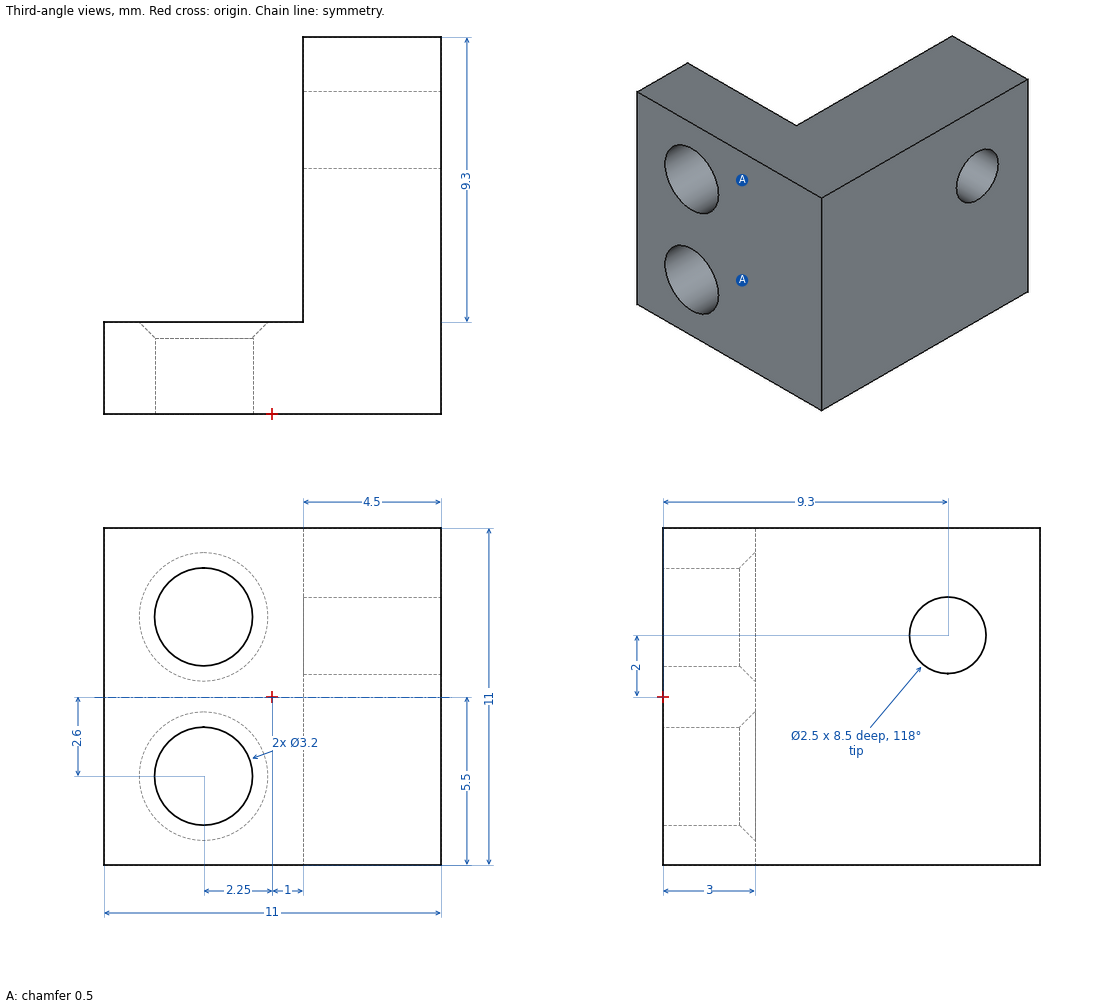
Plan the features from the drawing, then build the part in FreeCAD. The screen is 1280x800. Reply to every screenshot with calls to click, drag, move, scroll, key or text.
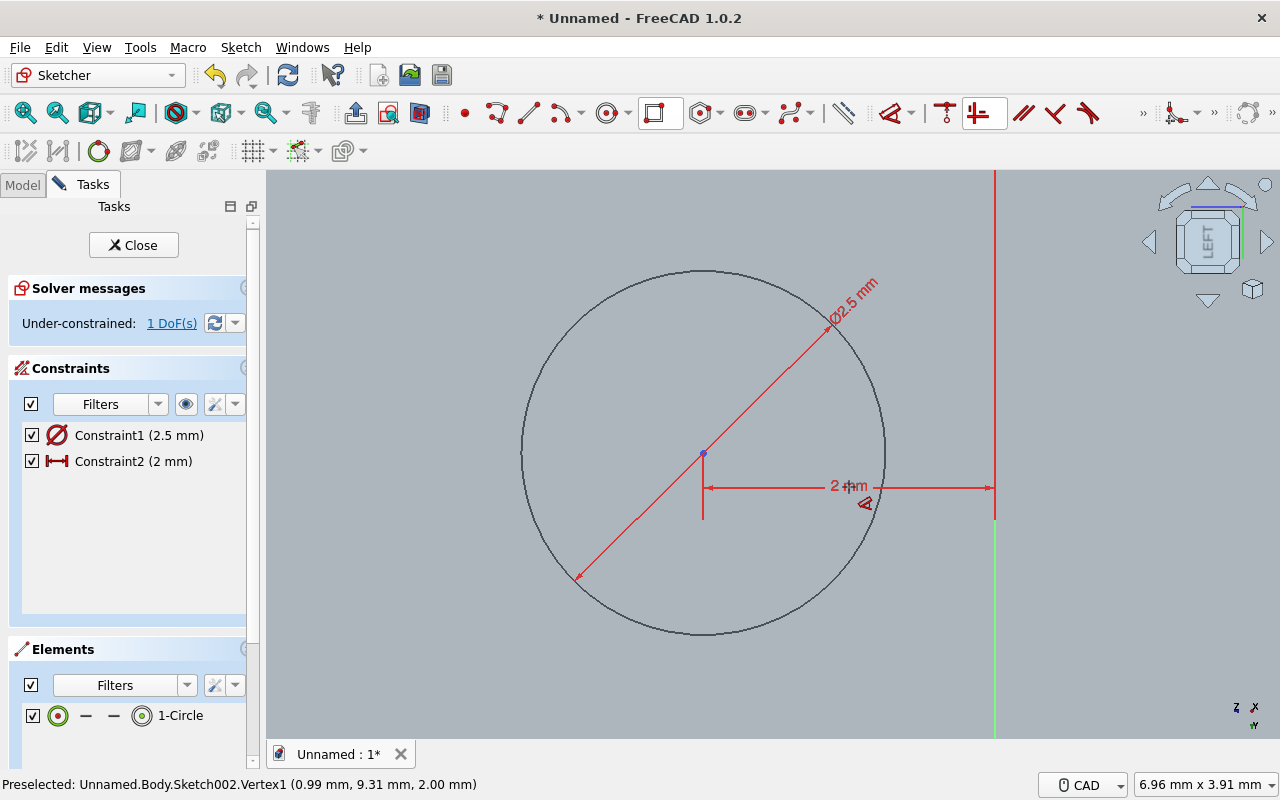
click(703, 453)
click(1029, 326)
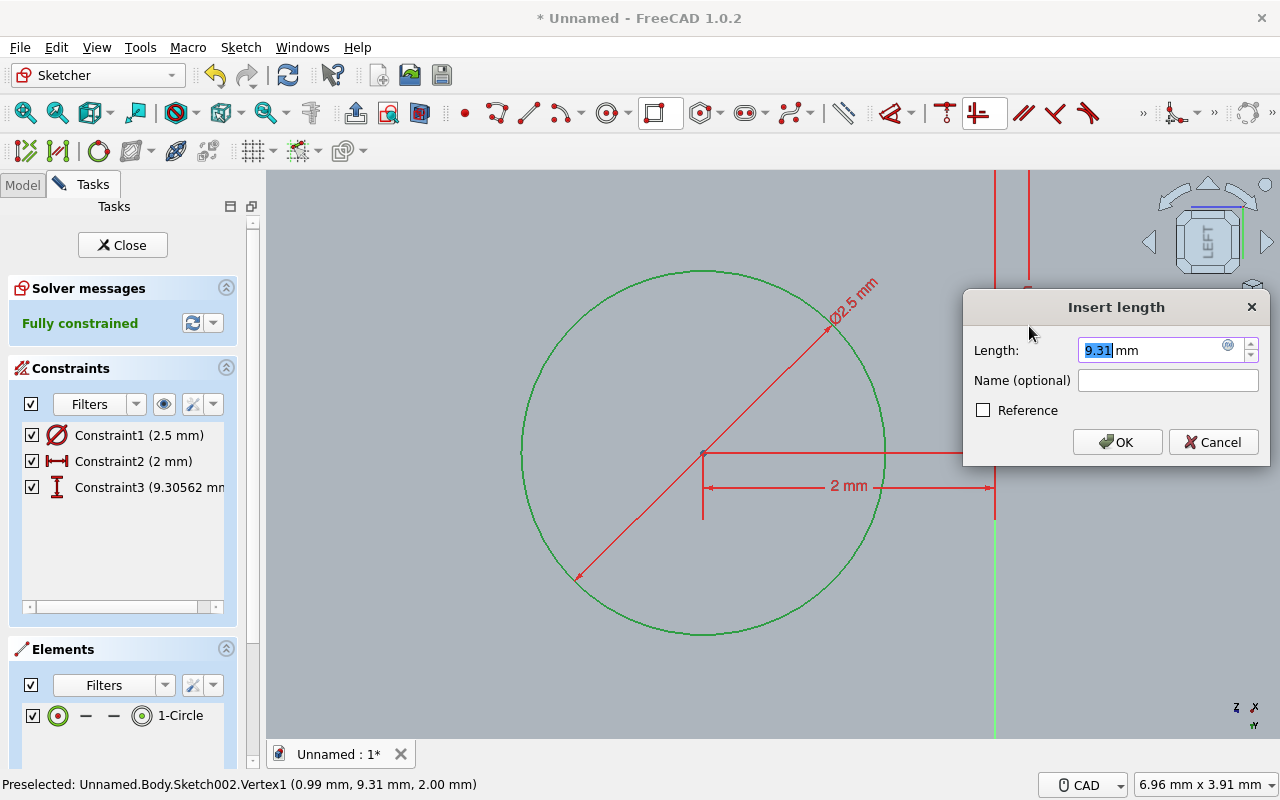
text(9.3)
key(Return)
key(Escape)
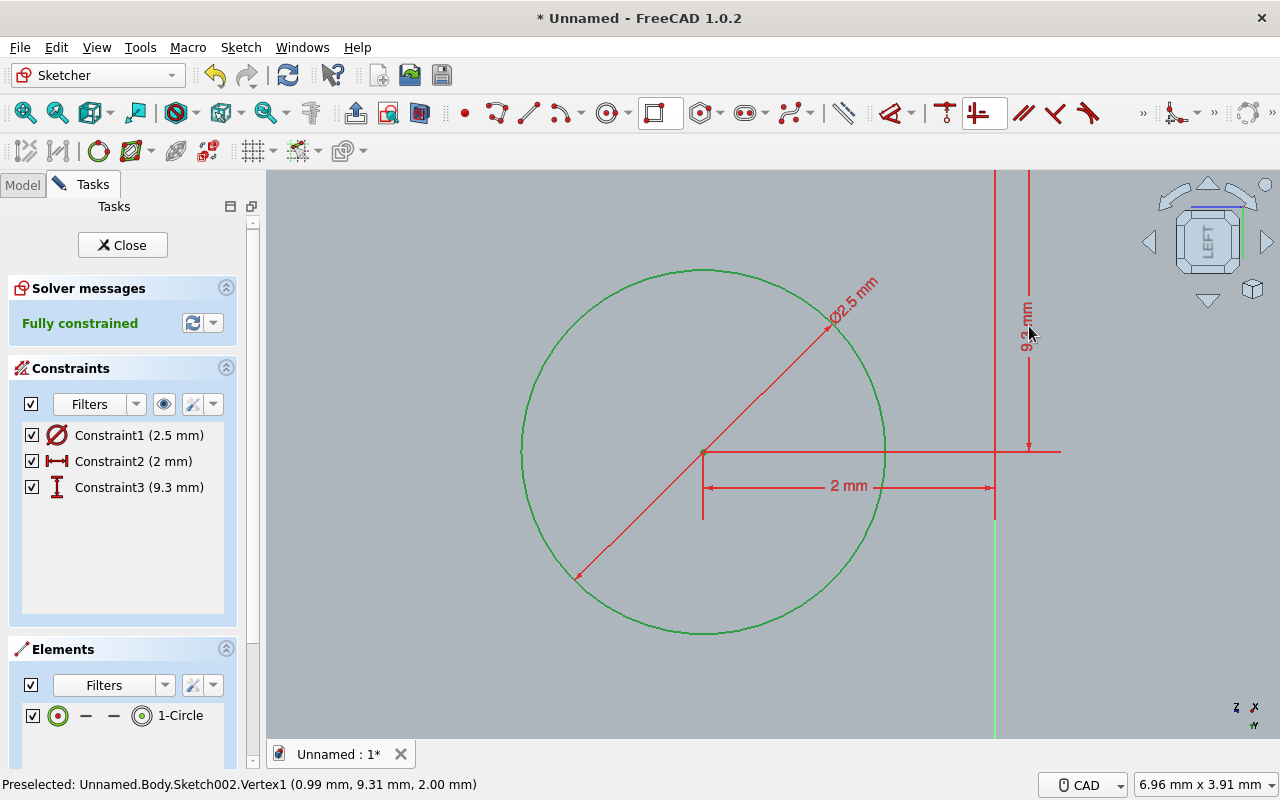
click(123, 245)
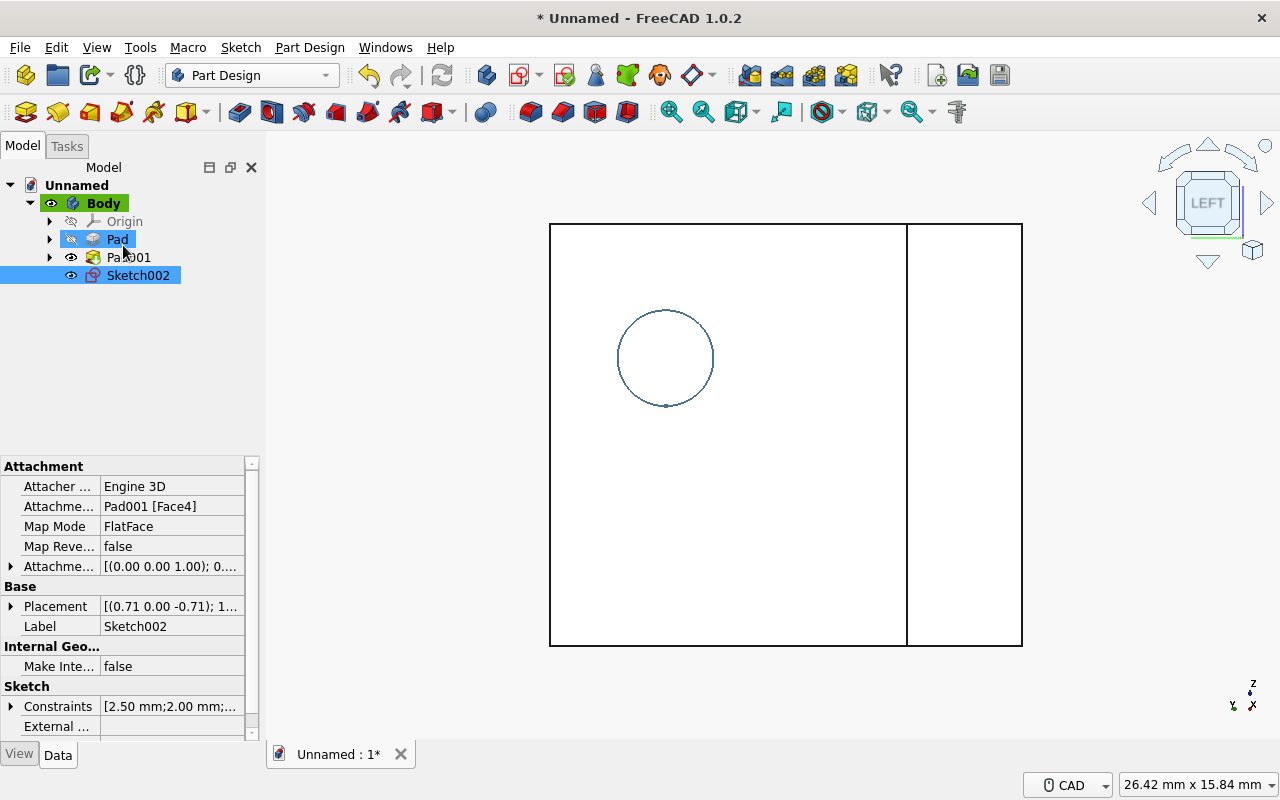
click(272, 112)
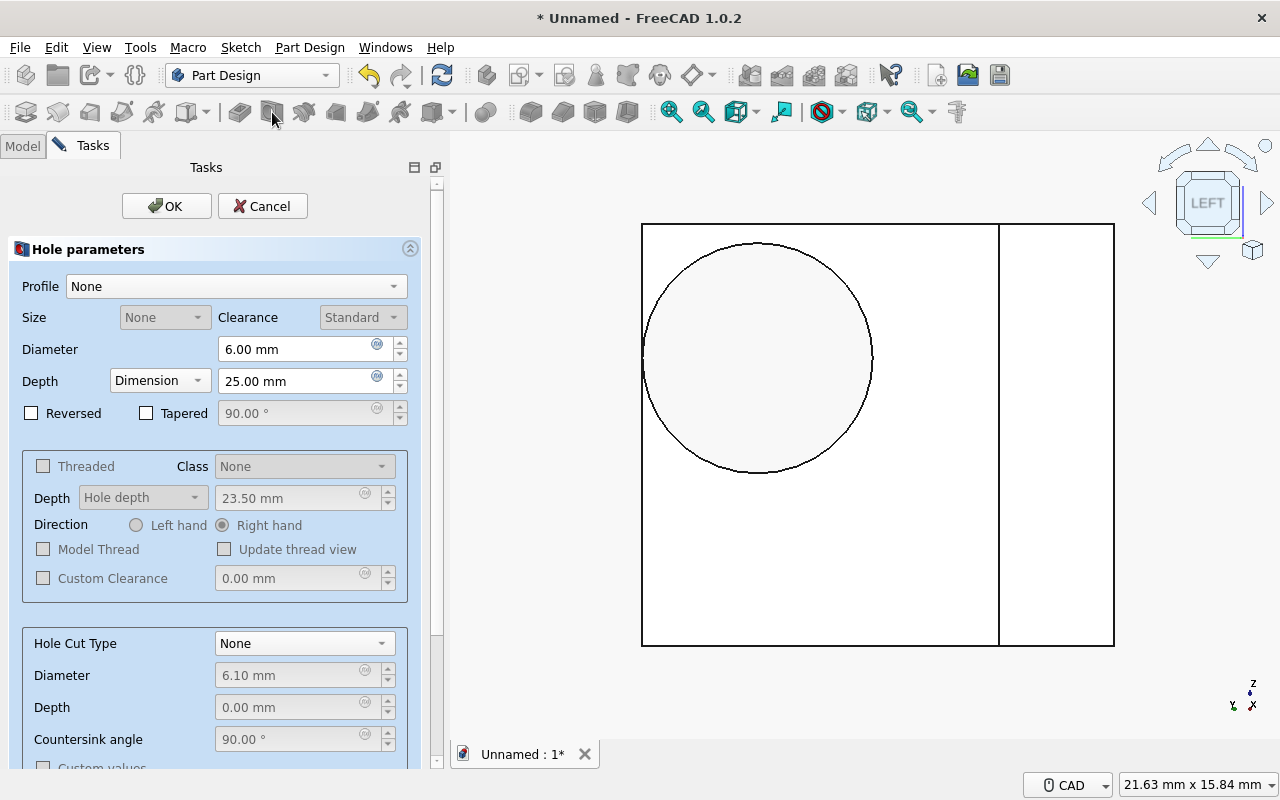
triple_click(305, 349)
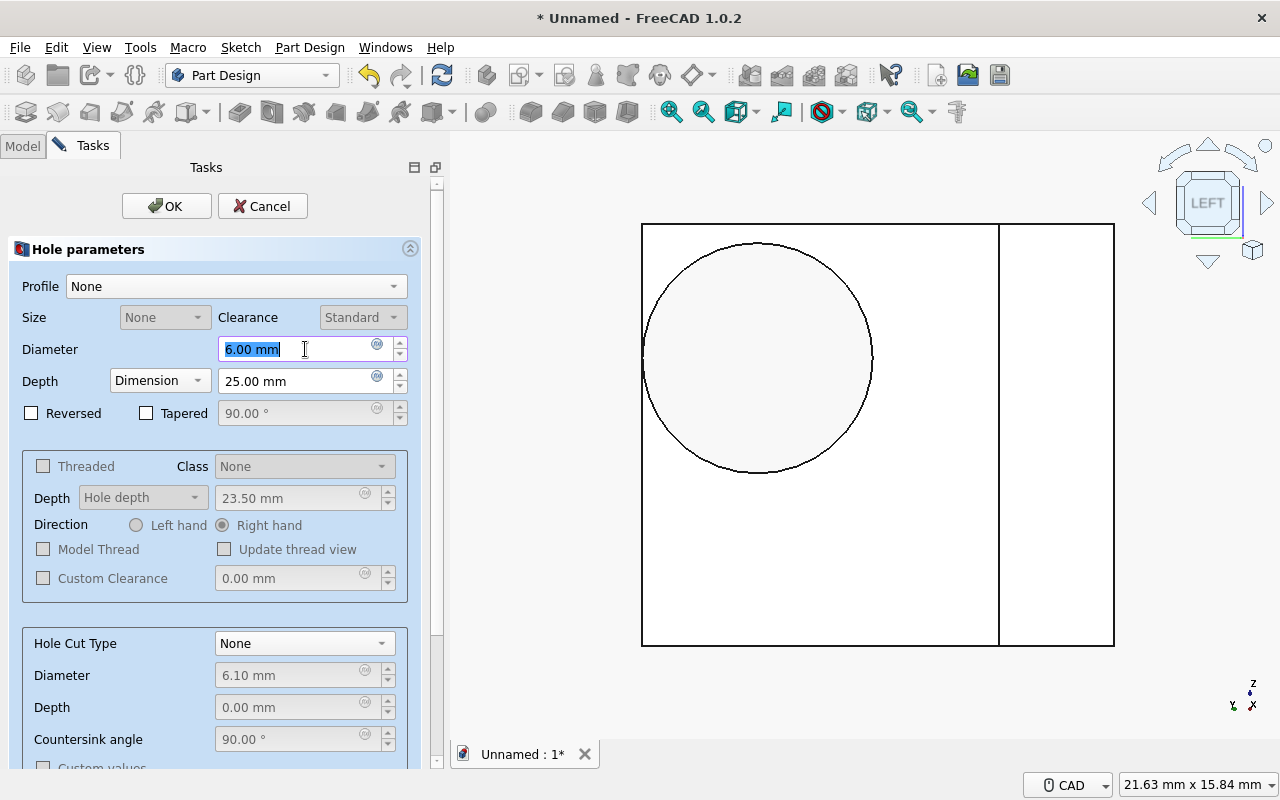
text(2.5)
key(Tab)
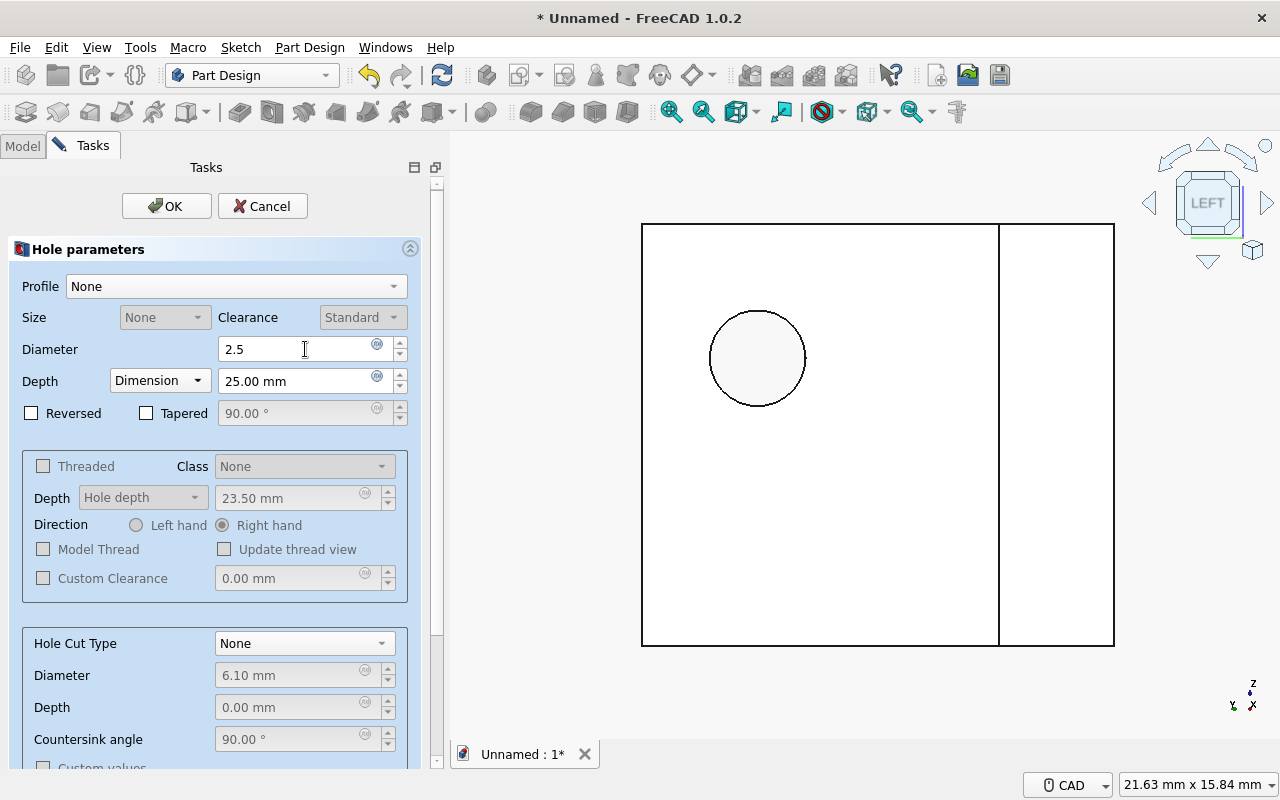
triple_click(305, 381)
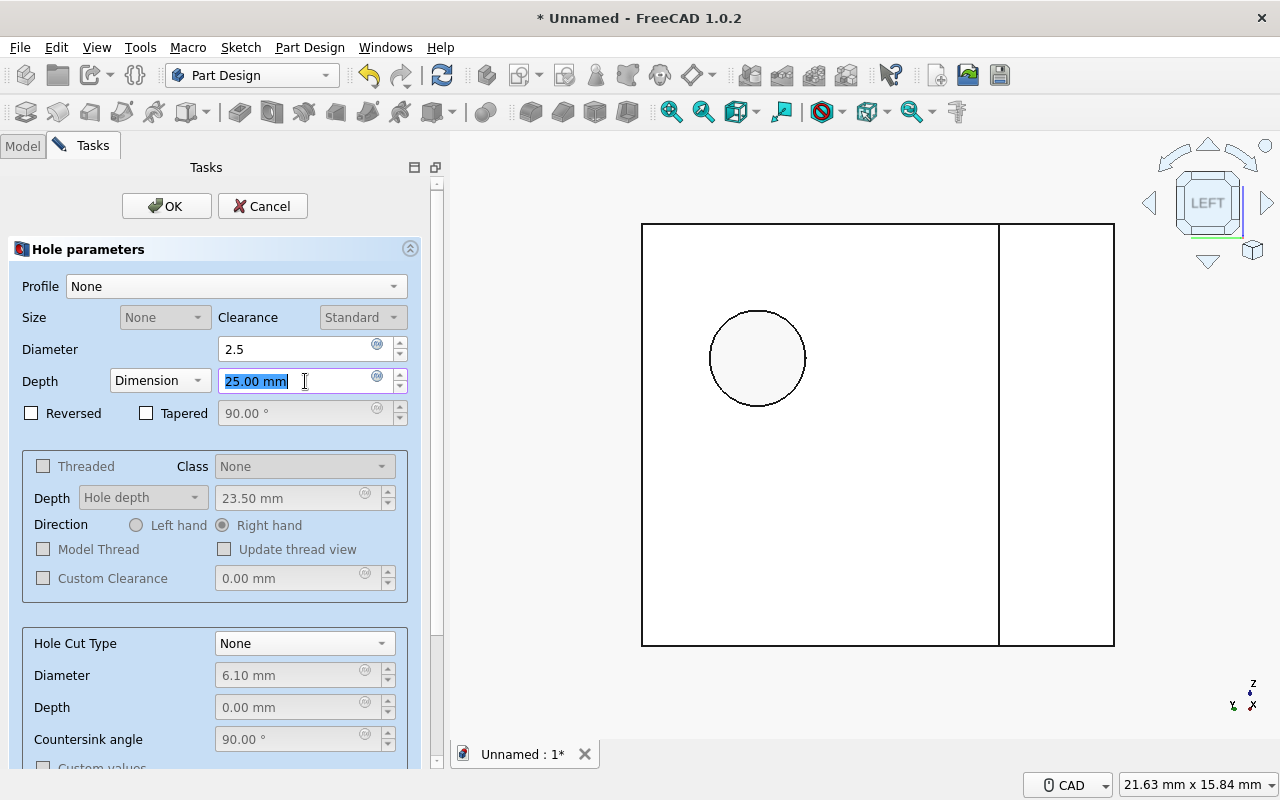
text(8.5)
key(Tab)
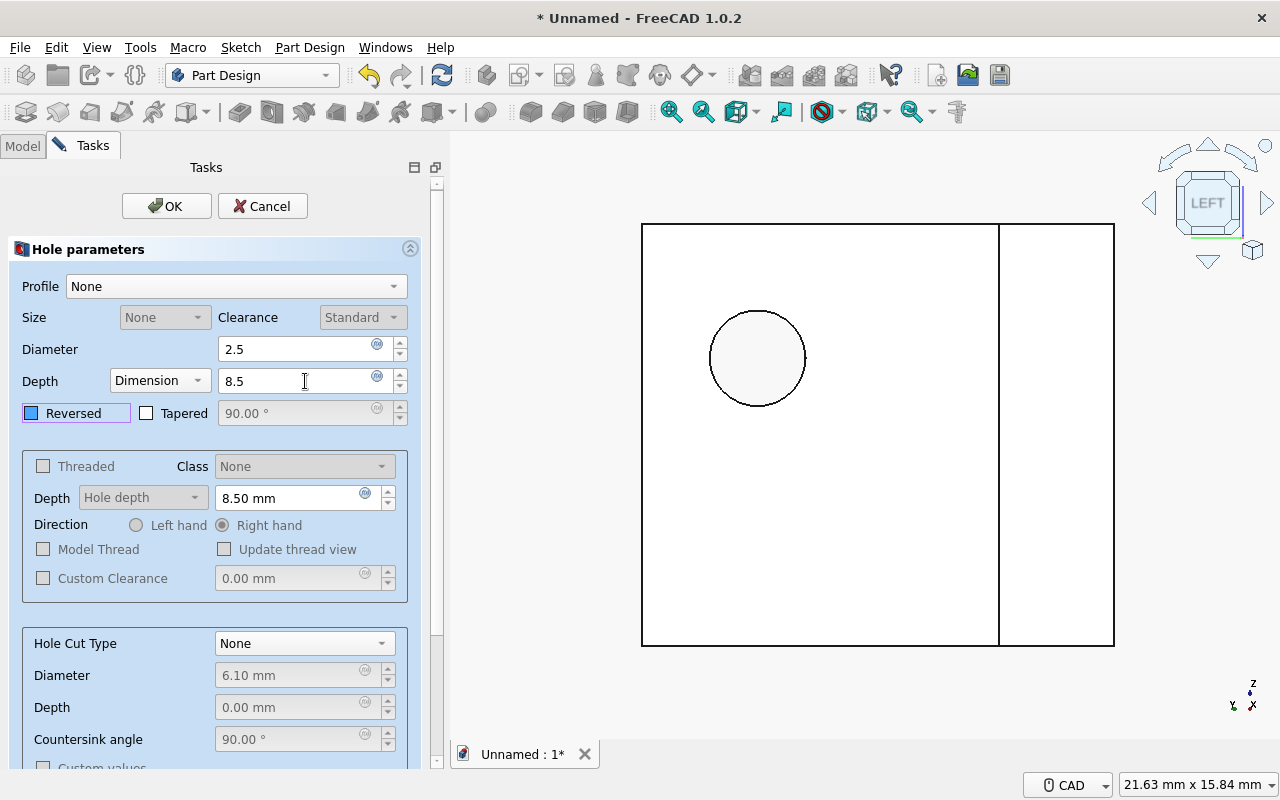
click(167, 206)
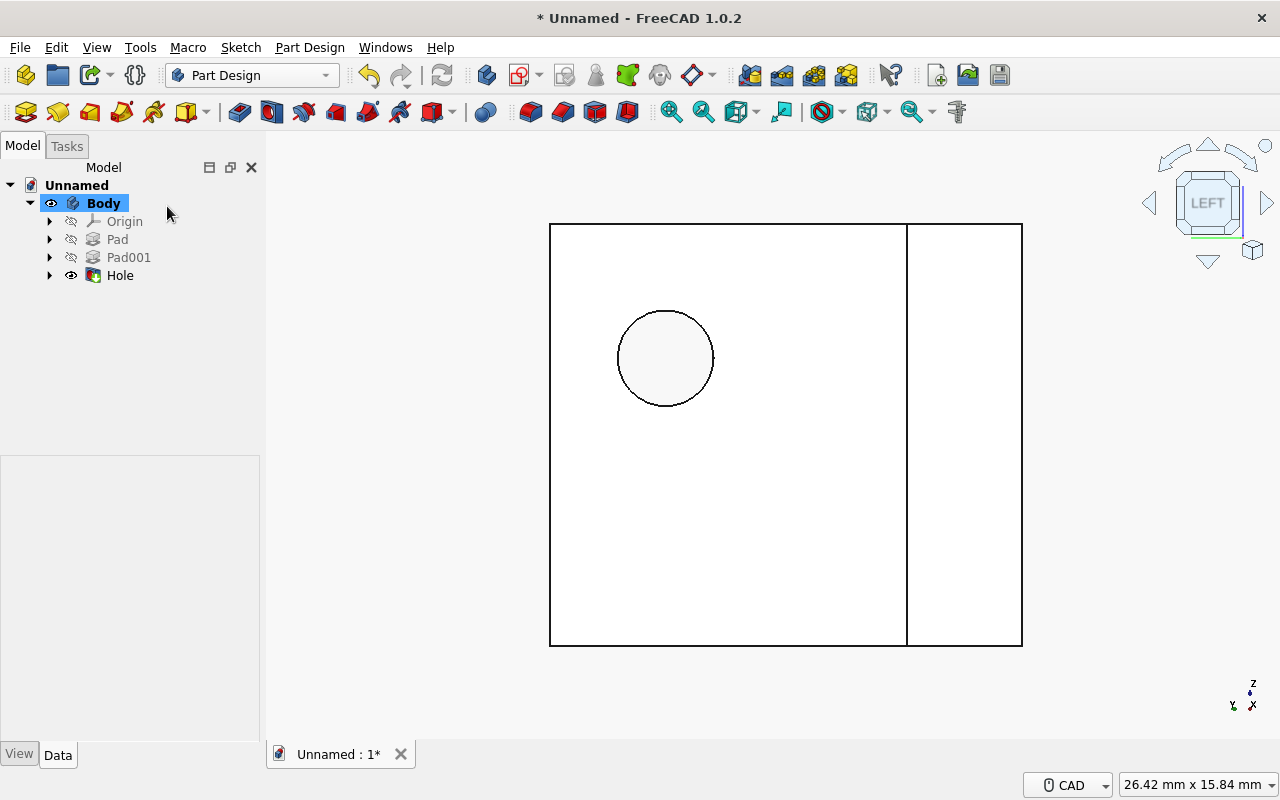
key(4)